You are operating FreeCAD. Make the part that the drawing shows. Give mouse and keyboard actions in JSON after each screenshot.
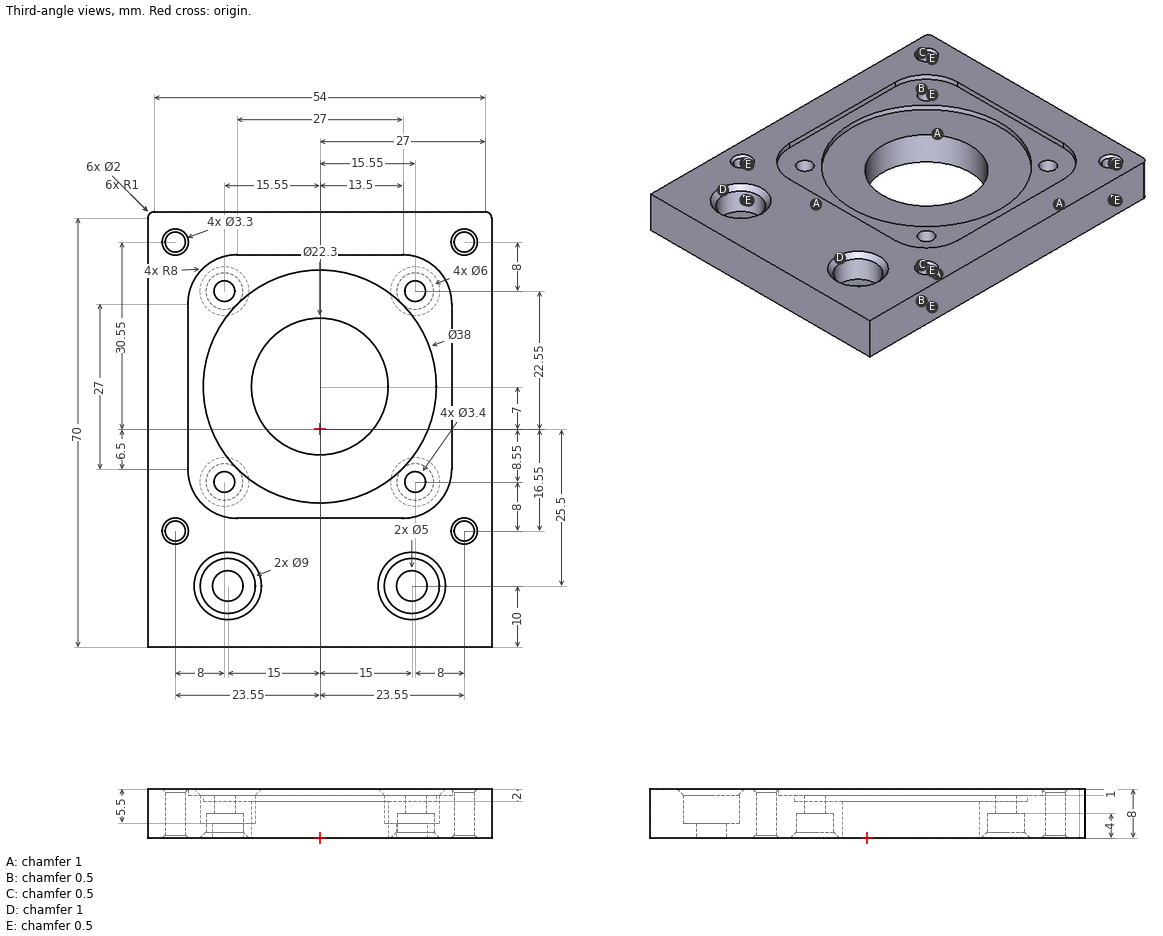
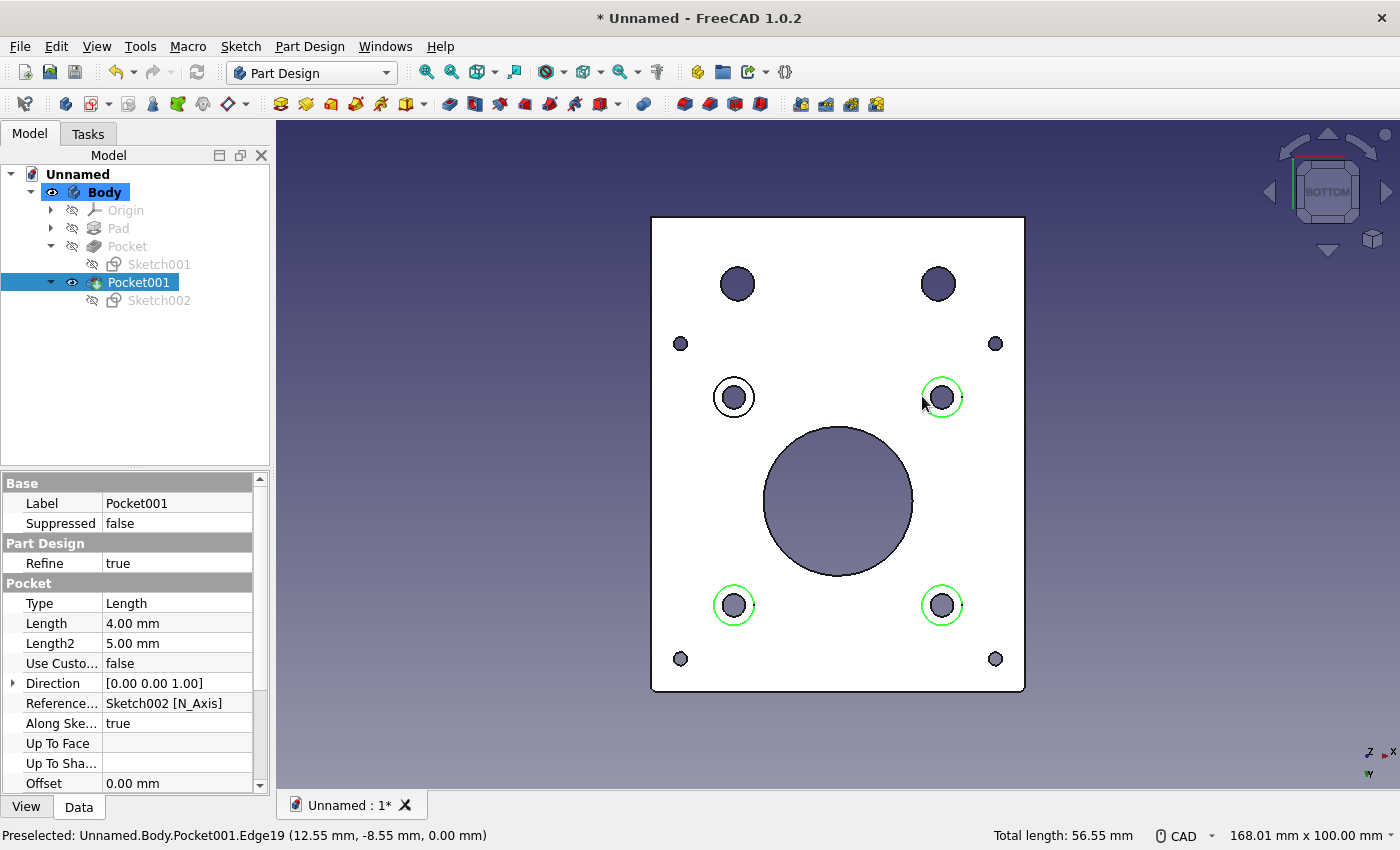
{"action": "left_click", "coordinate": [714, 396], "text": "ctrl"}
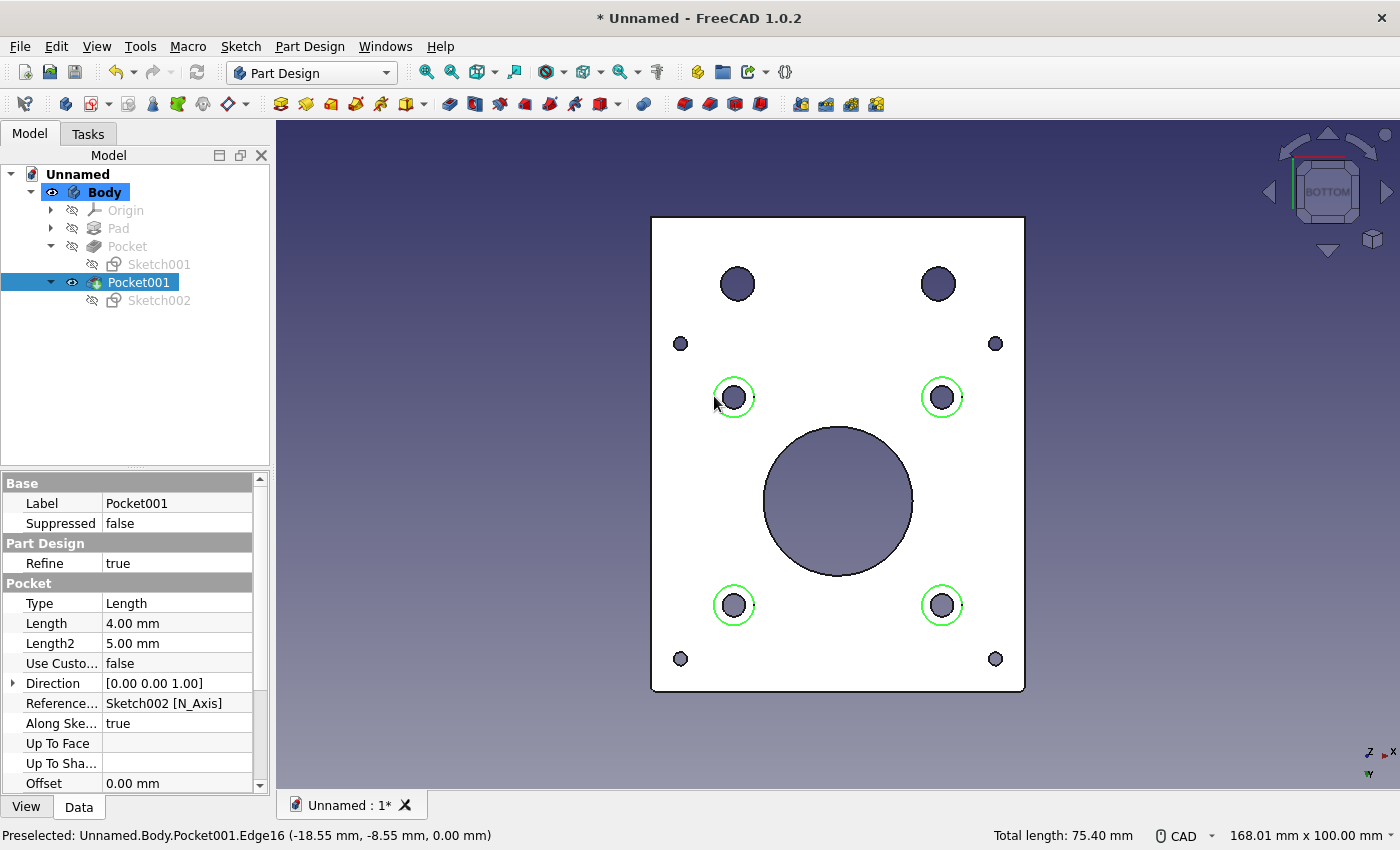
{"action": "left_click", "coordinate": [710, 104]}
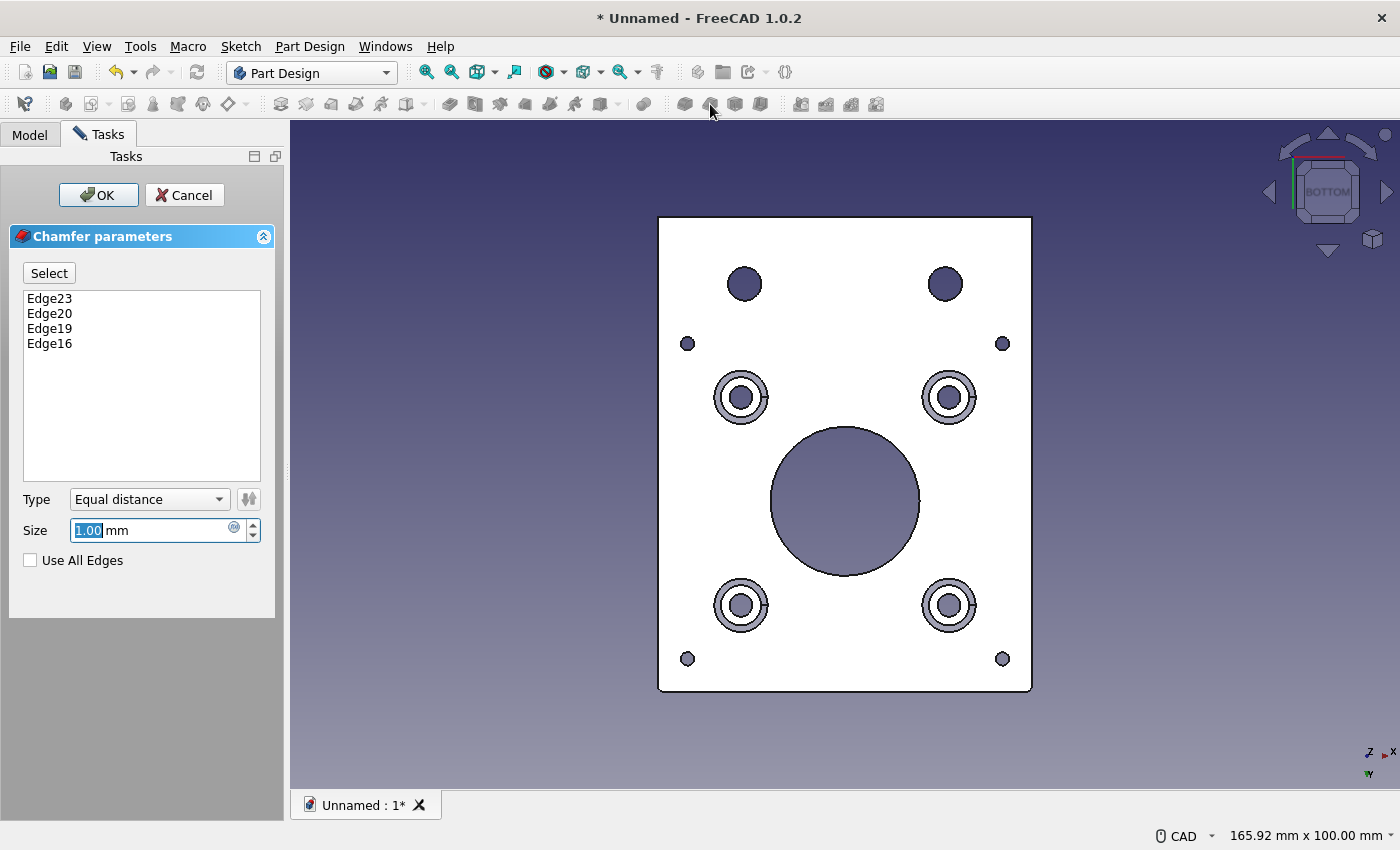
{"action": "type", "text": "1"}
{"action": "key", "text": "Tab"}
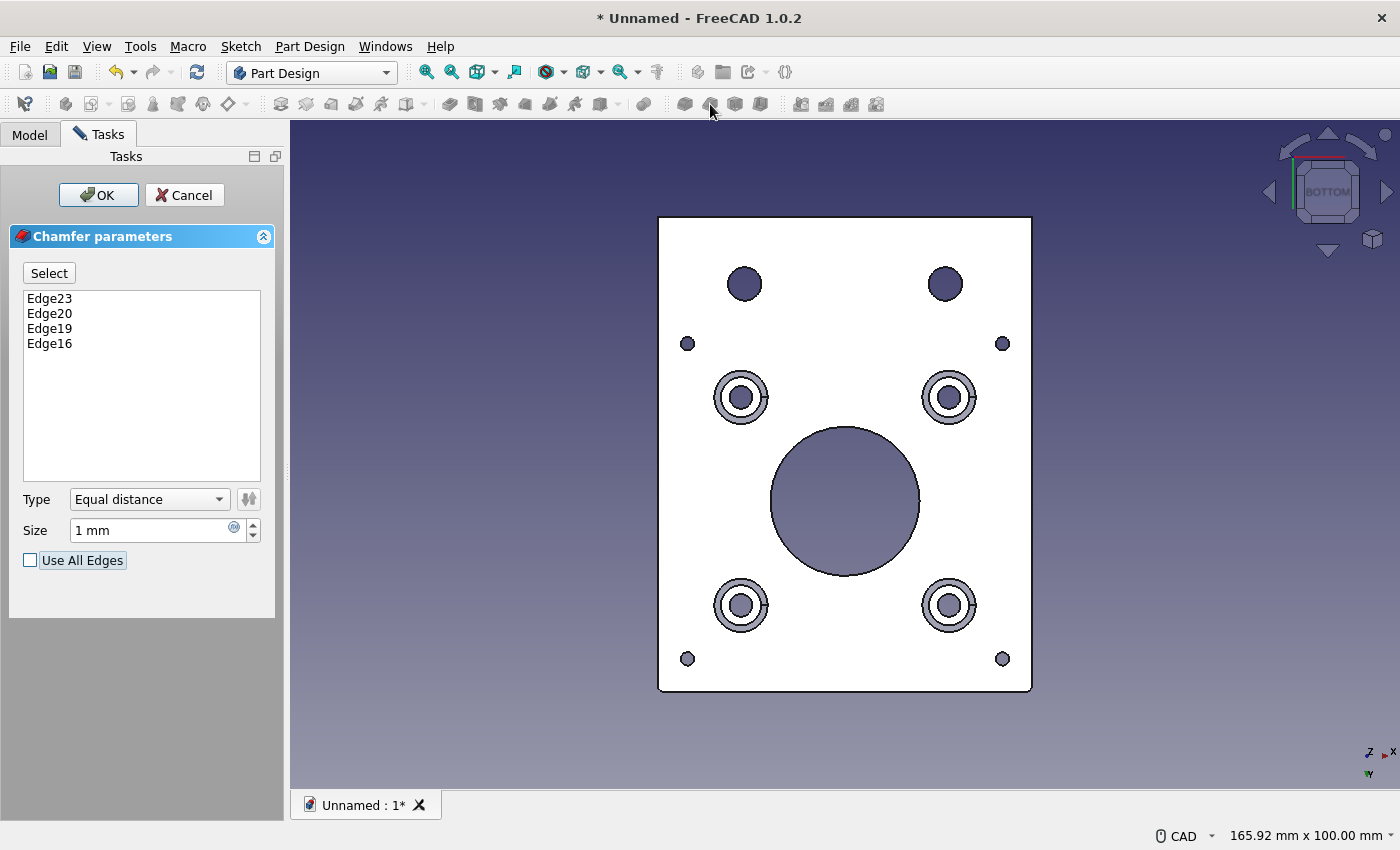
{"action": "left_click", "coordinate": [99, 195]}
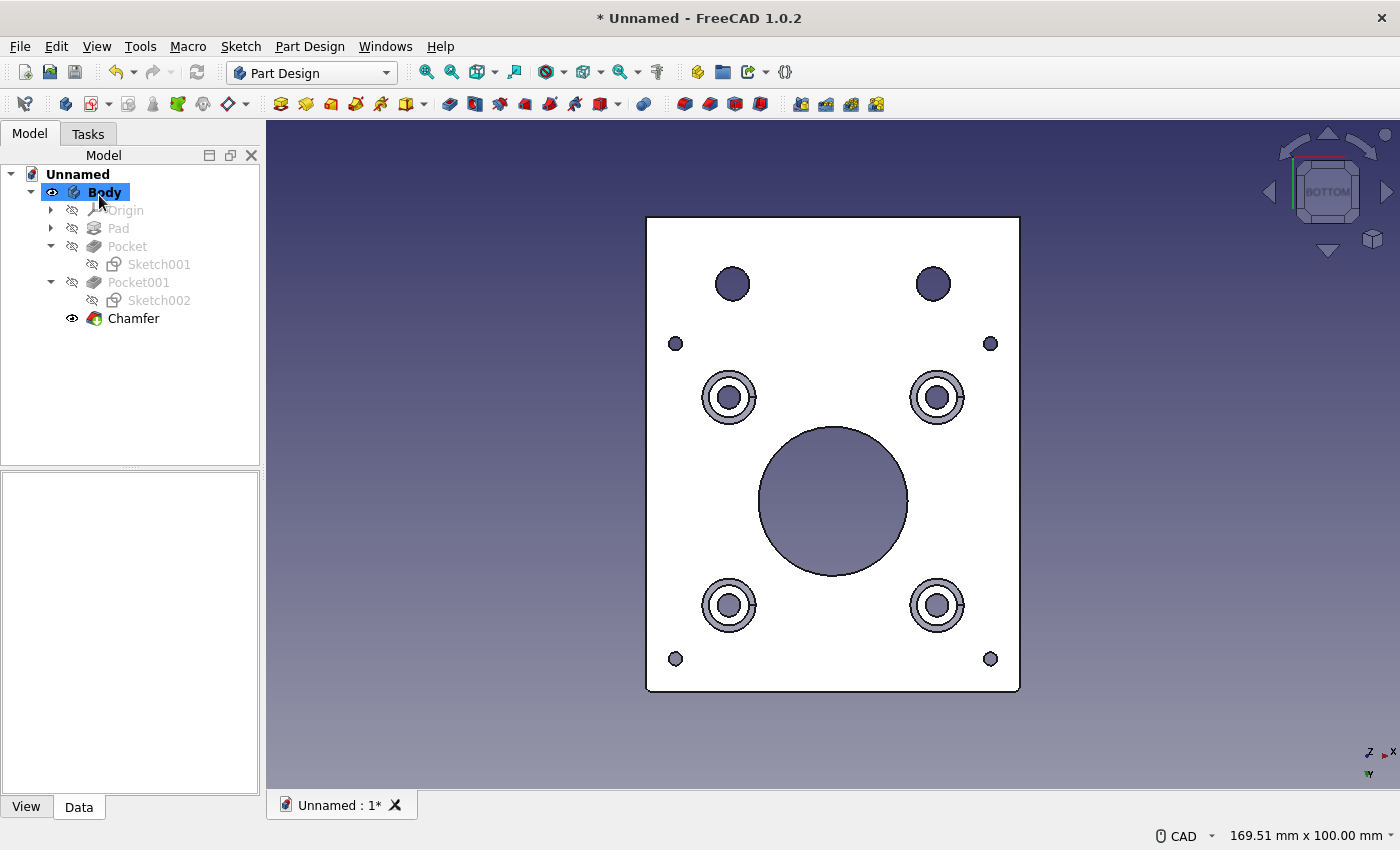
{"action": "left_click", "coordinate": [669, 658]}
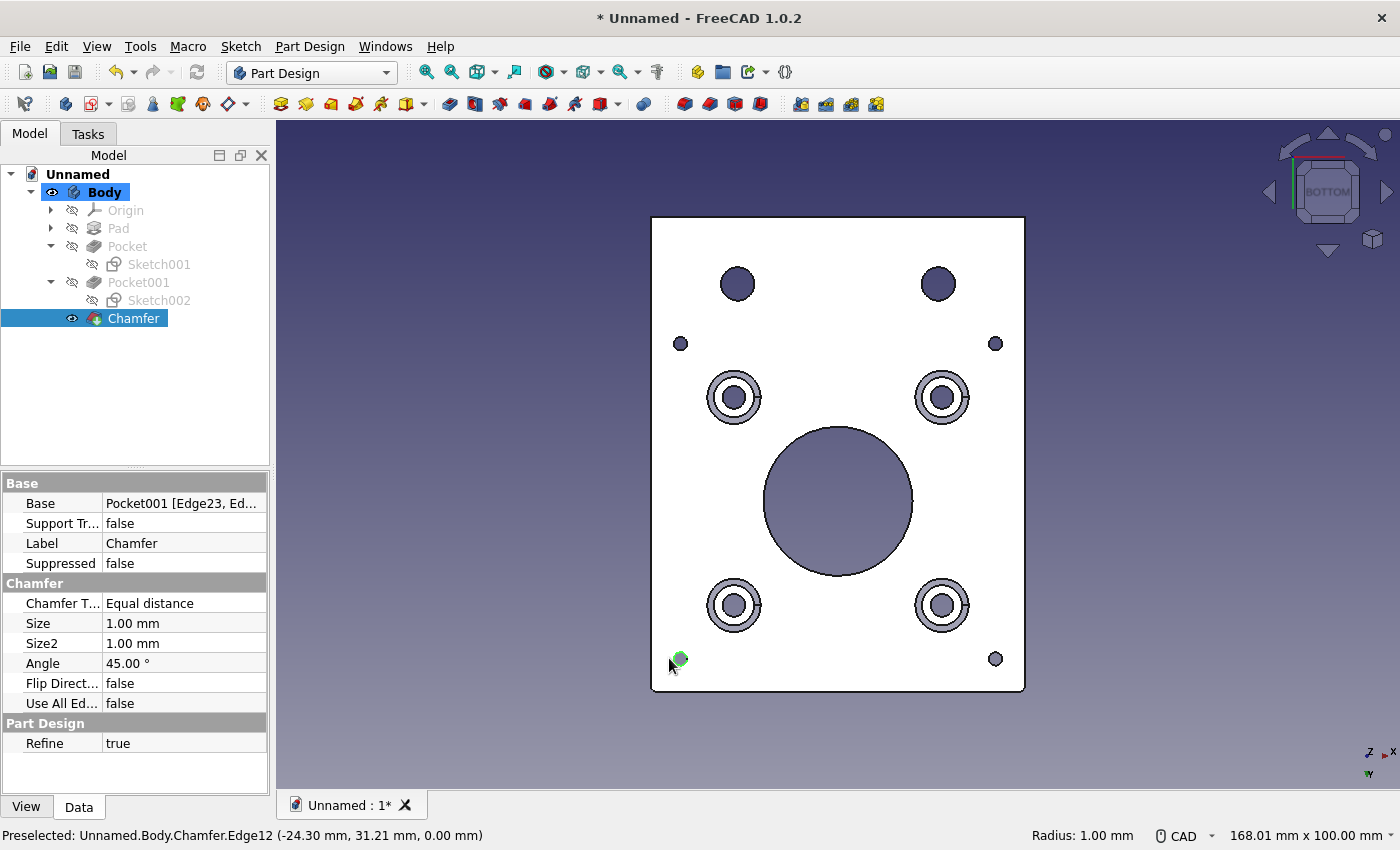
{"action": "left_click", "coordinate": [989, 658], "text": "ctrl"}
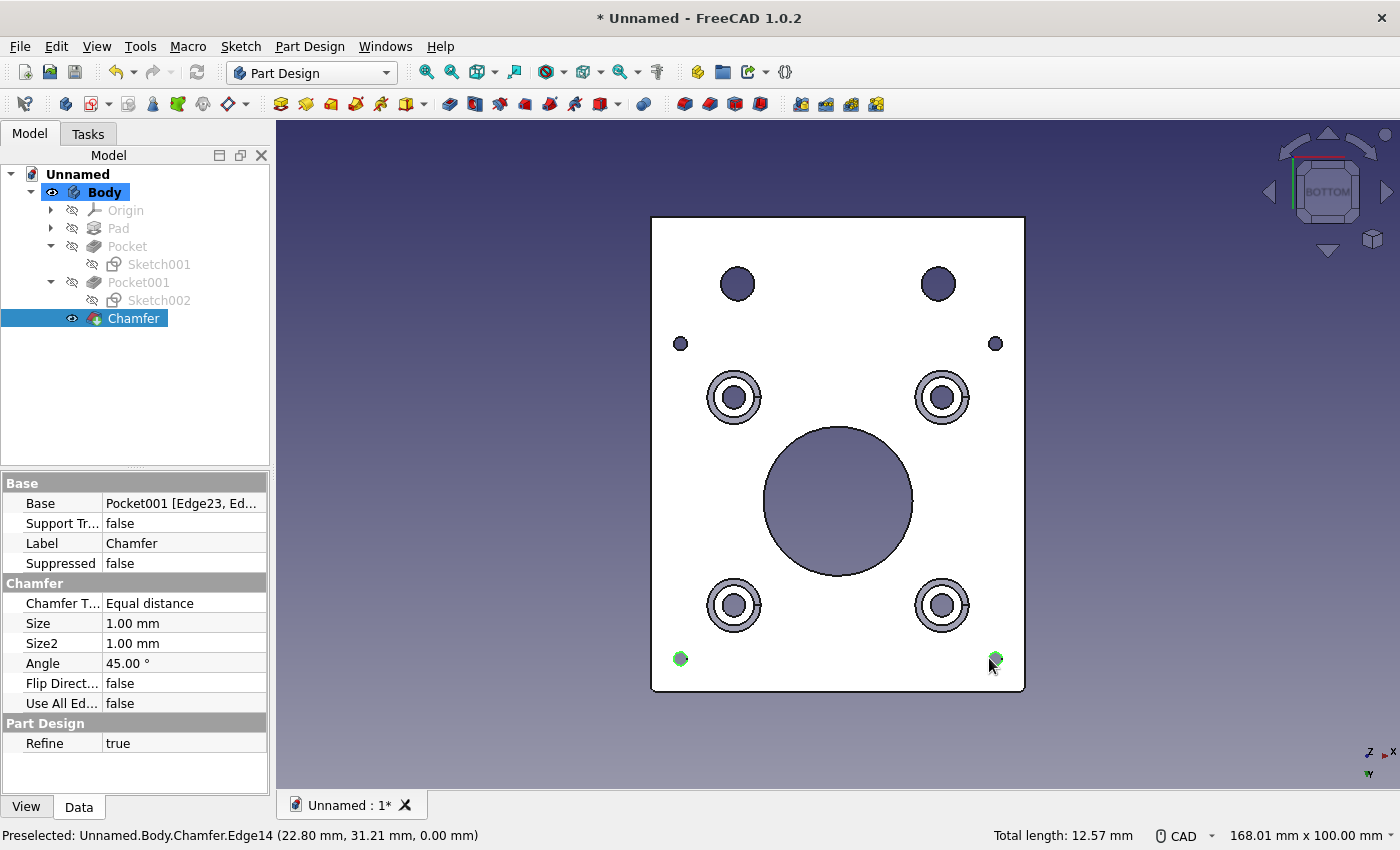
{"action": "left_click", "coordinate": [674, 343], "text": "ctrl"}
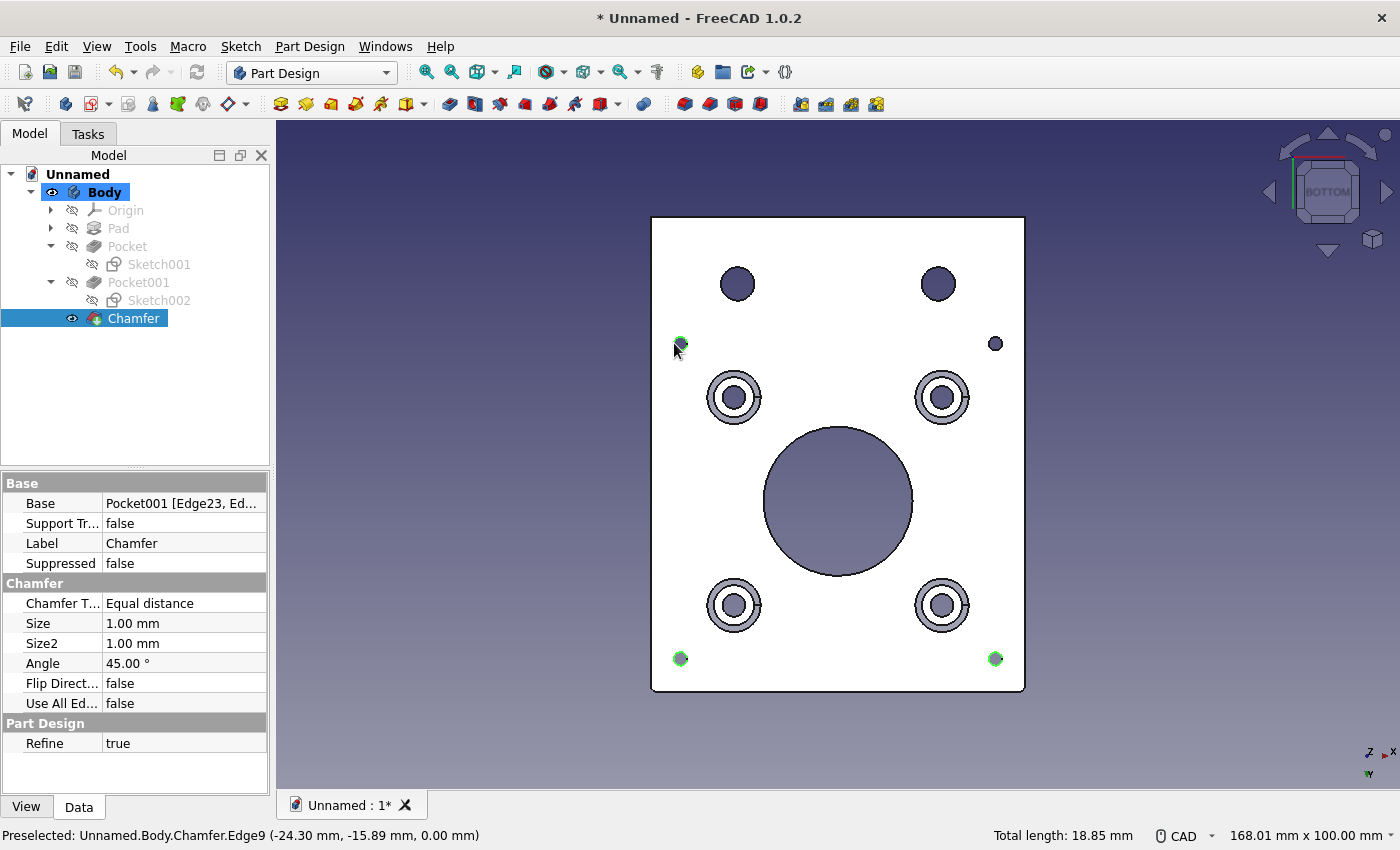
{"action": "left_click", "coordinate": [989, 343], "text": "ctrl"}